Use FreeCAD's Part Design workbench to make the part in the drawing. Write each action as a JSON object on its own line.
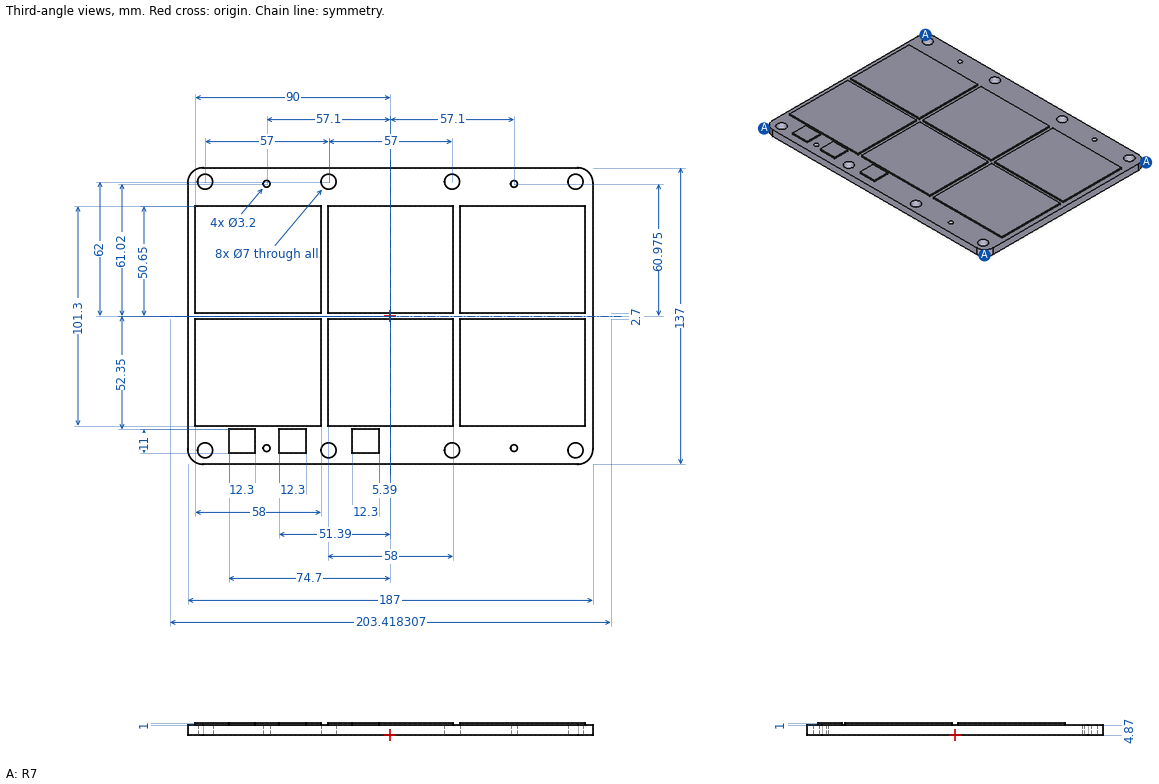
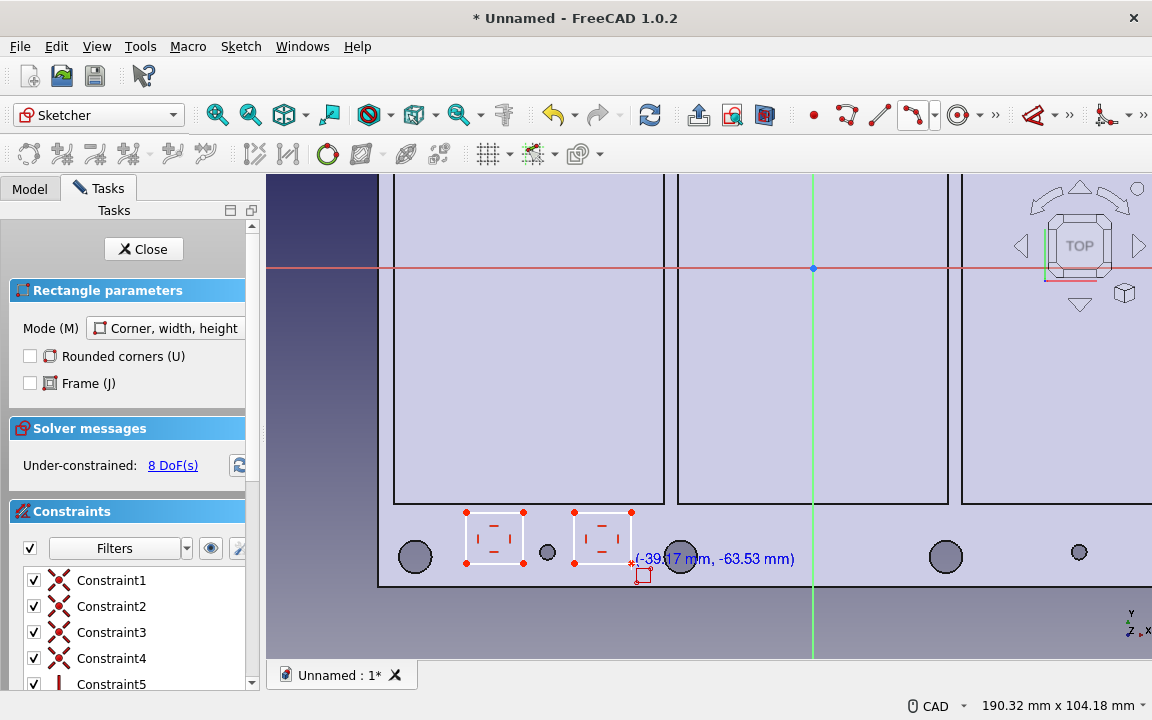
{"action": "left_click", "coordinate": [731, 512]}
{"action": "left_click", "coordinate": [788, 563]}
{"action": "key", "text": "Escape"}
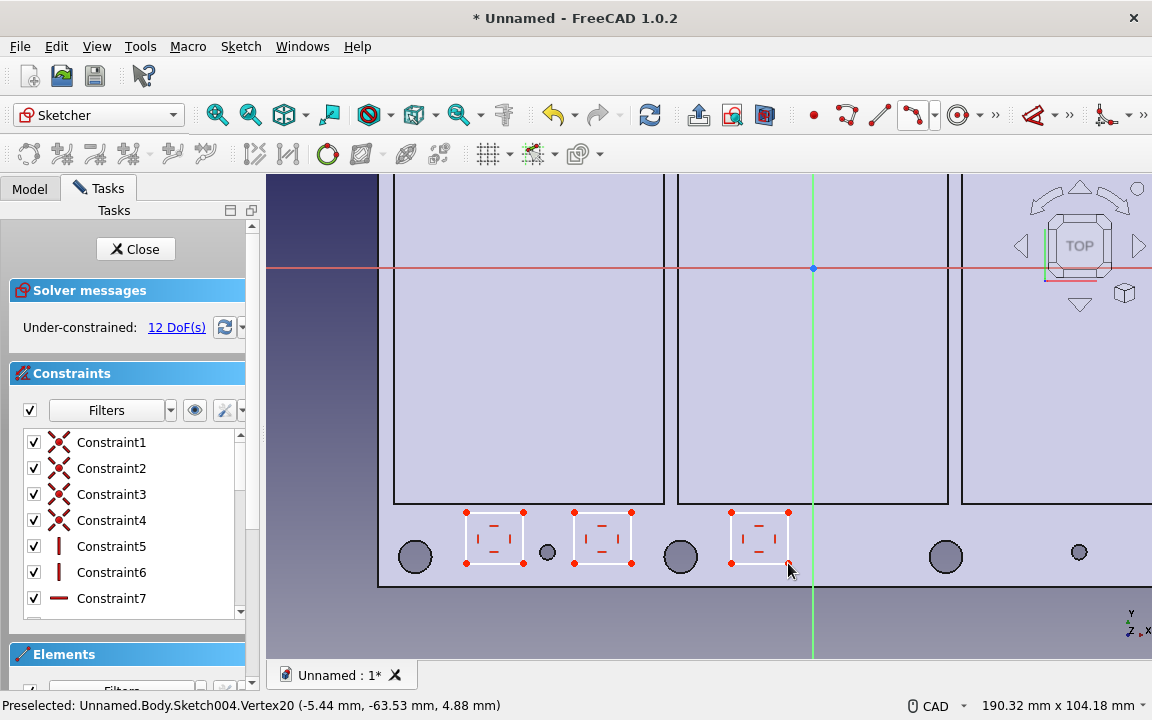
{"action": "key", "text": "d"}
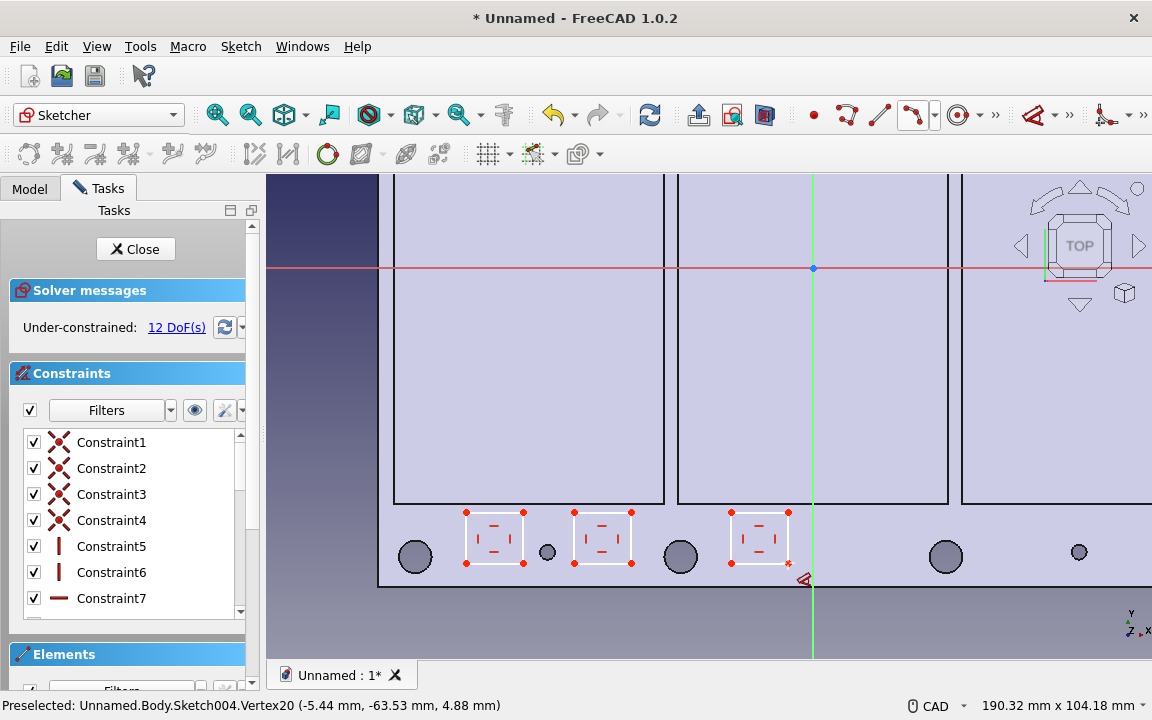
{"action": "left_click", "coordinate": [466, 528]}
{"action": "left_click", "coordinate": [432, 539]}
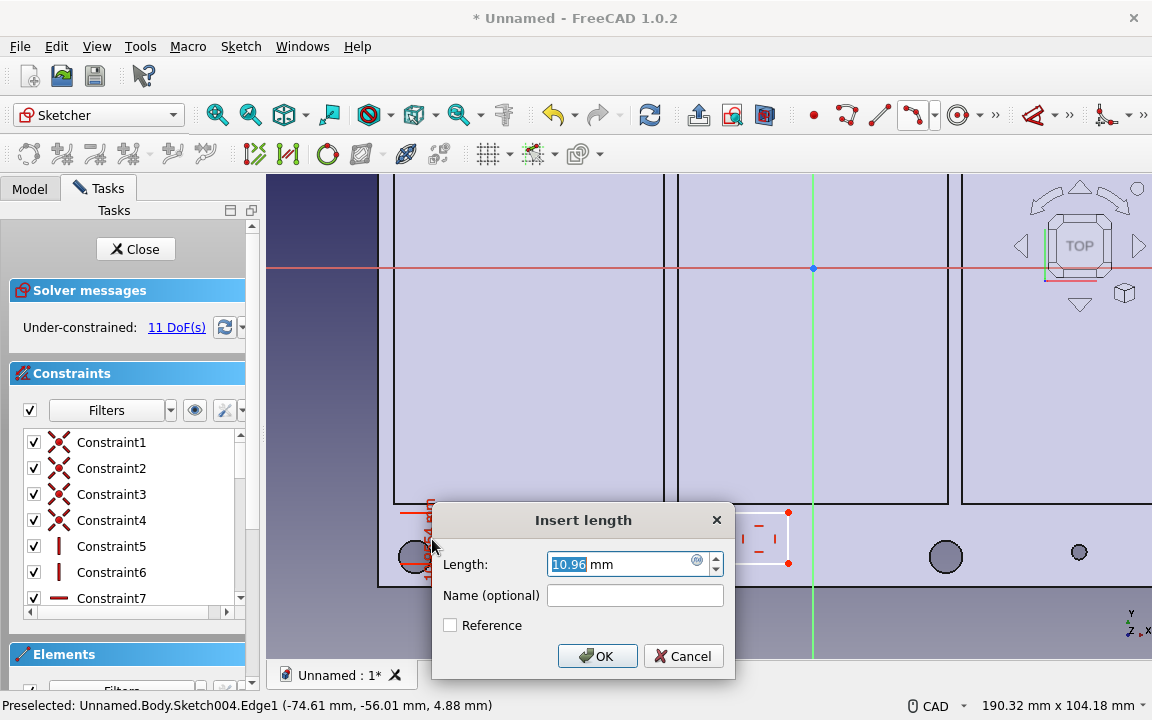
{"action": "type", "text": "11"}
{"action": "key", "text": "Return"}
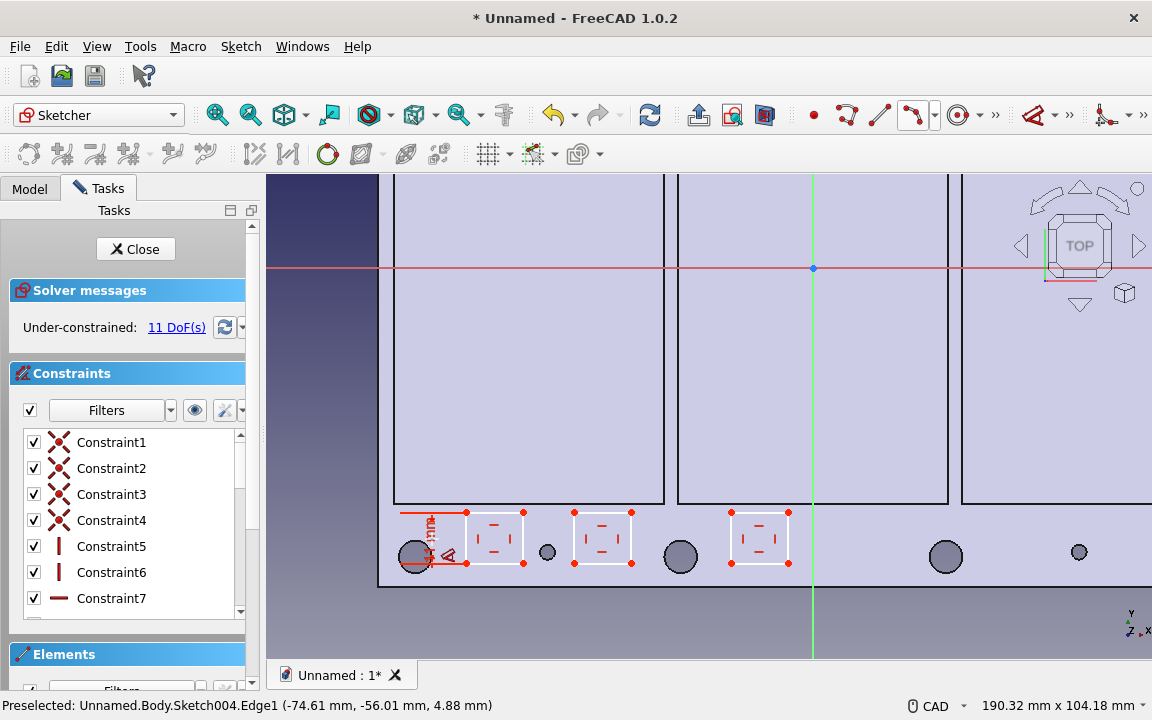
{"action": "left_click", "coordinate": [574, 528]}
{"action": "left_click", "coordinate": [540, 539]}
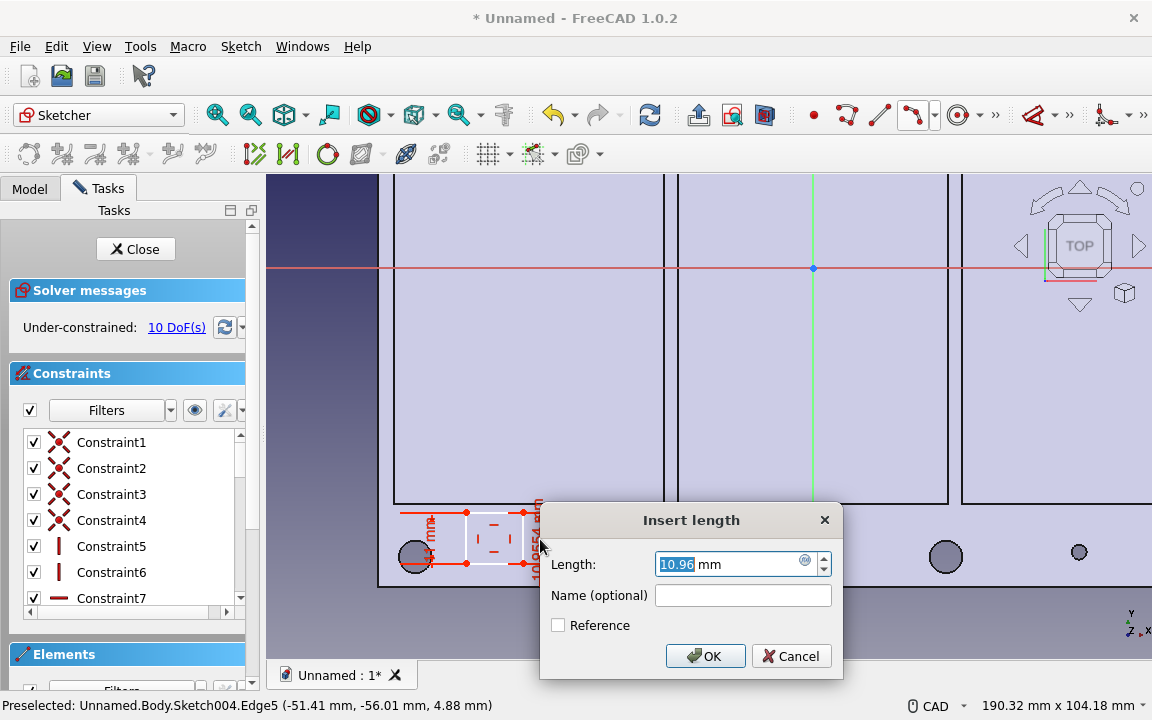
{"action": "type", "text": "11"}
{"action": "key", "text": "Return"}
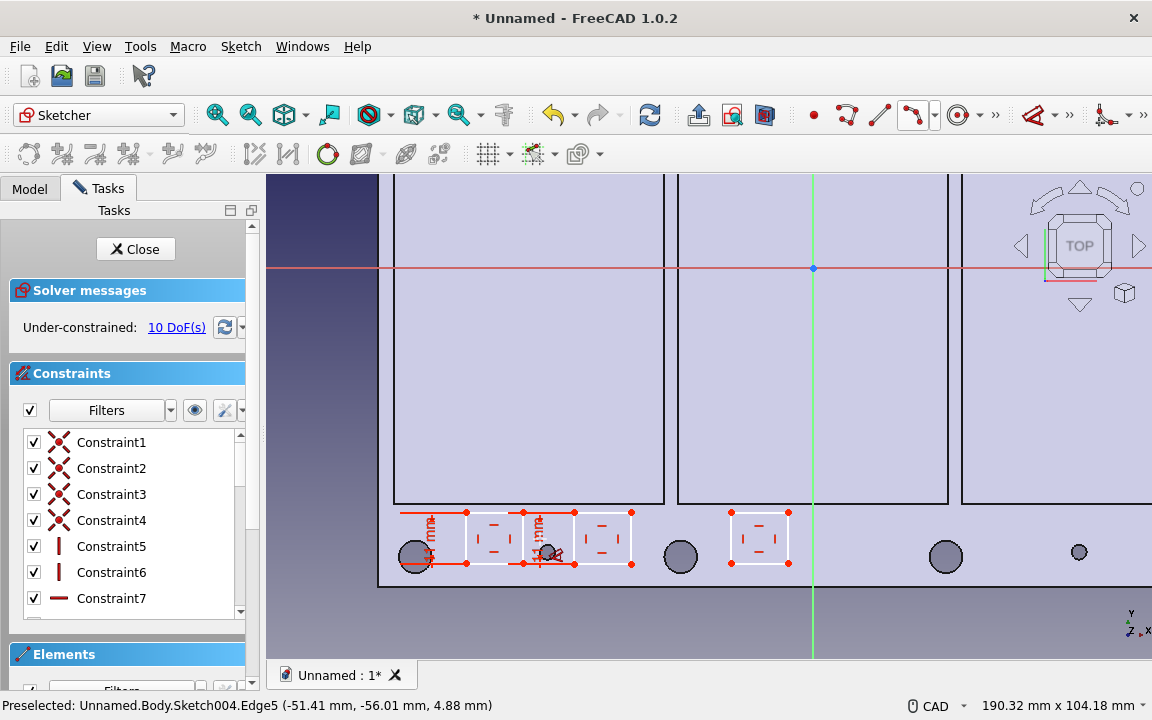
{"action": "left_click", "coordinate": [731, 528]}
{"action": "left_click", "coordinate": [765, 539]}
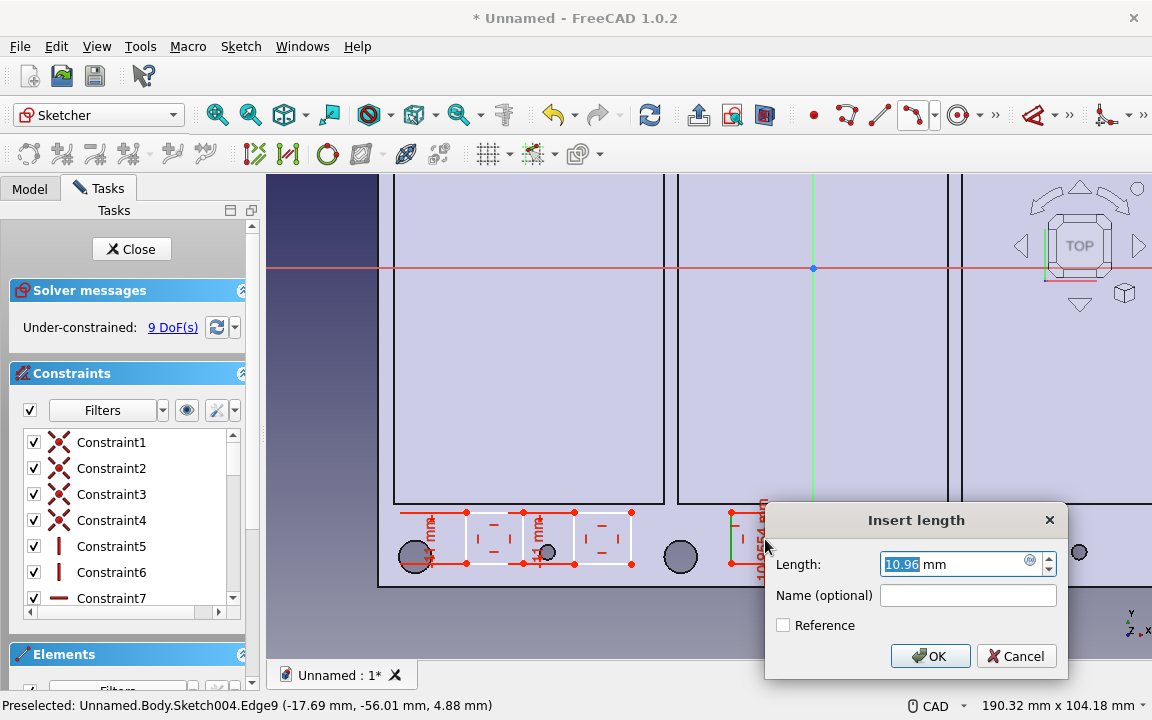
{"action": "type", "text": "11"}
{"action": "key", "text": "Return"}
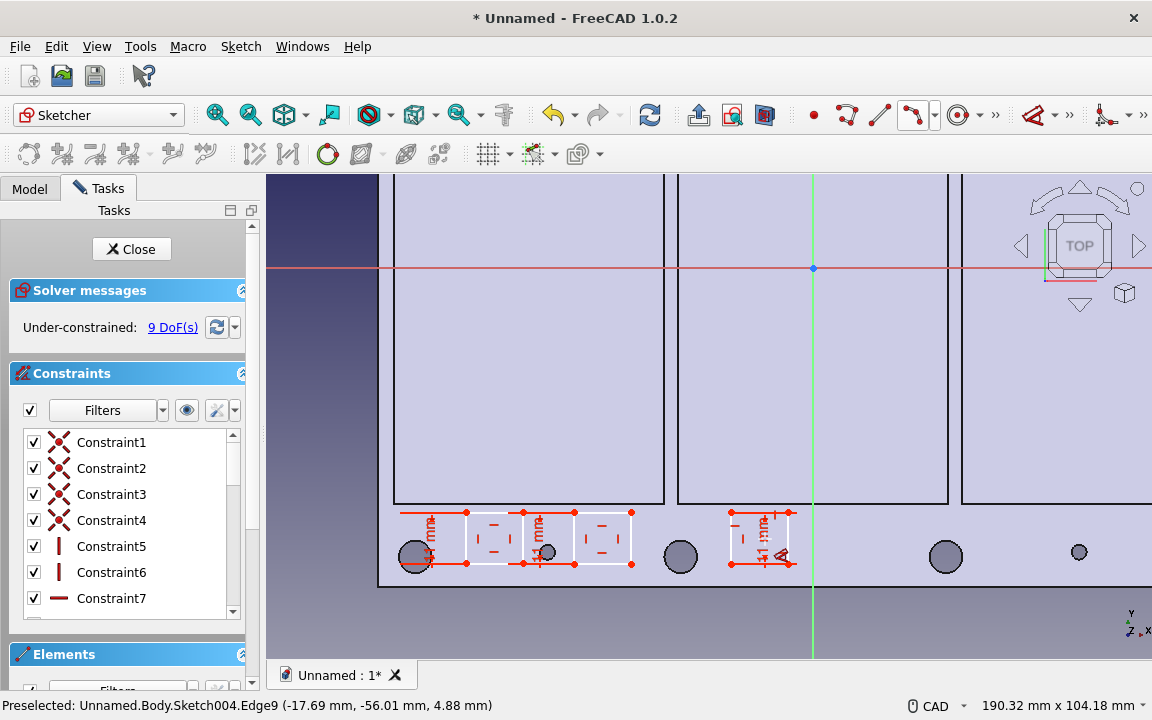
{"action": "left_click", "coordinate": [483, 564]}
{"action": "left_click", "coordinate": [495, 598]}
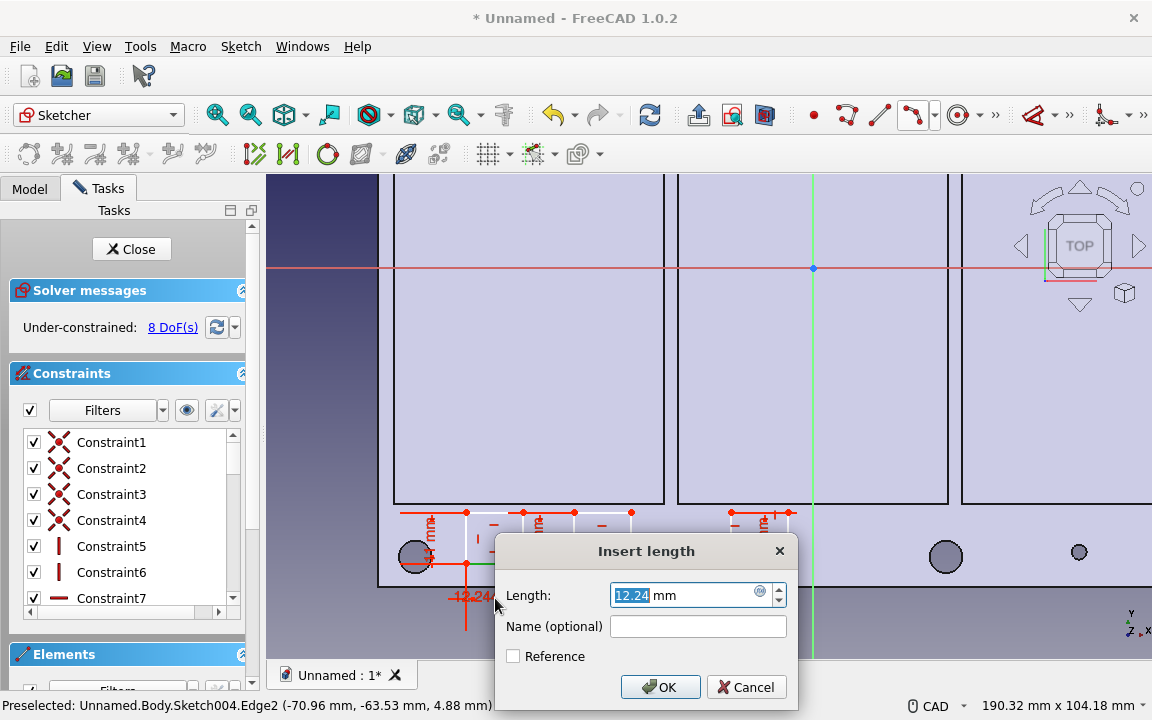
{"action": "type", "text": "12.3"}
{"action": "key", "text": "Return"}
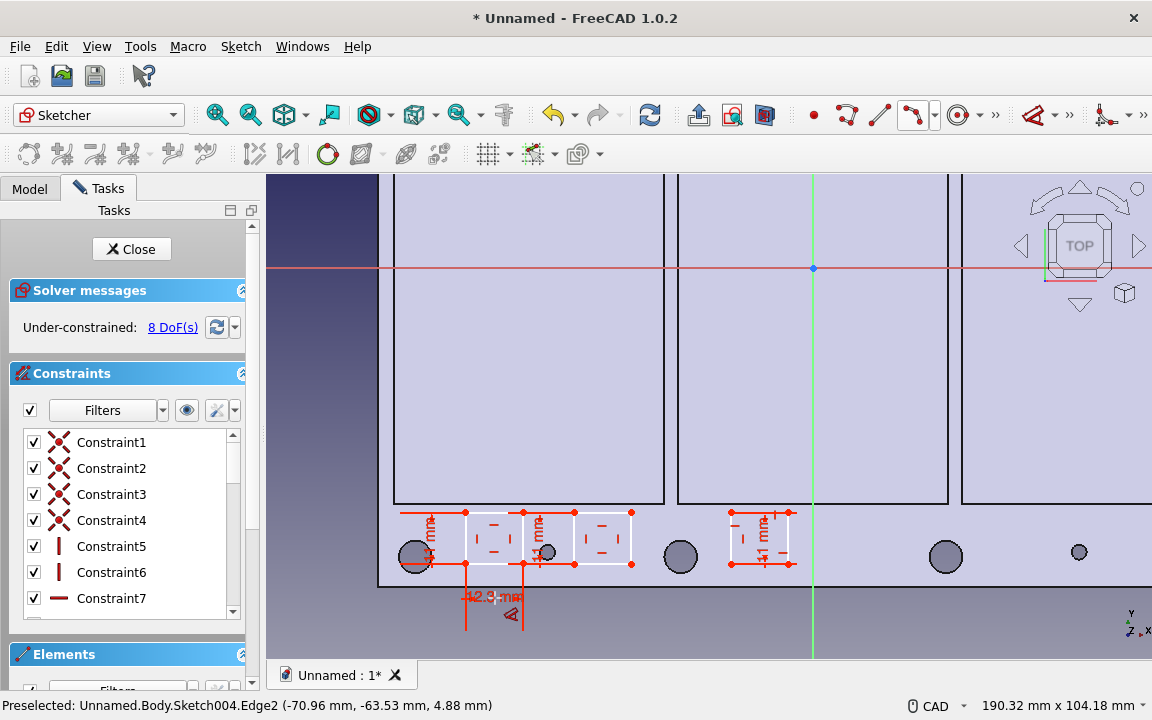
{"action": "left_click", "coordinate": [591, 564]}
{"action": "left_click", "coordinate": [602, 598]}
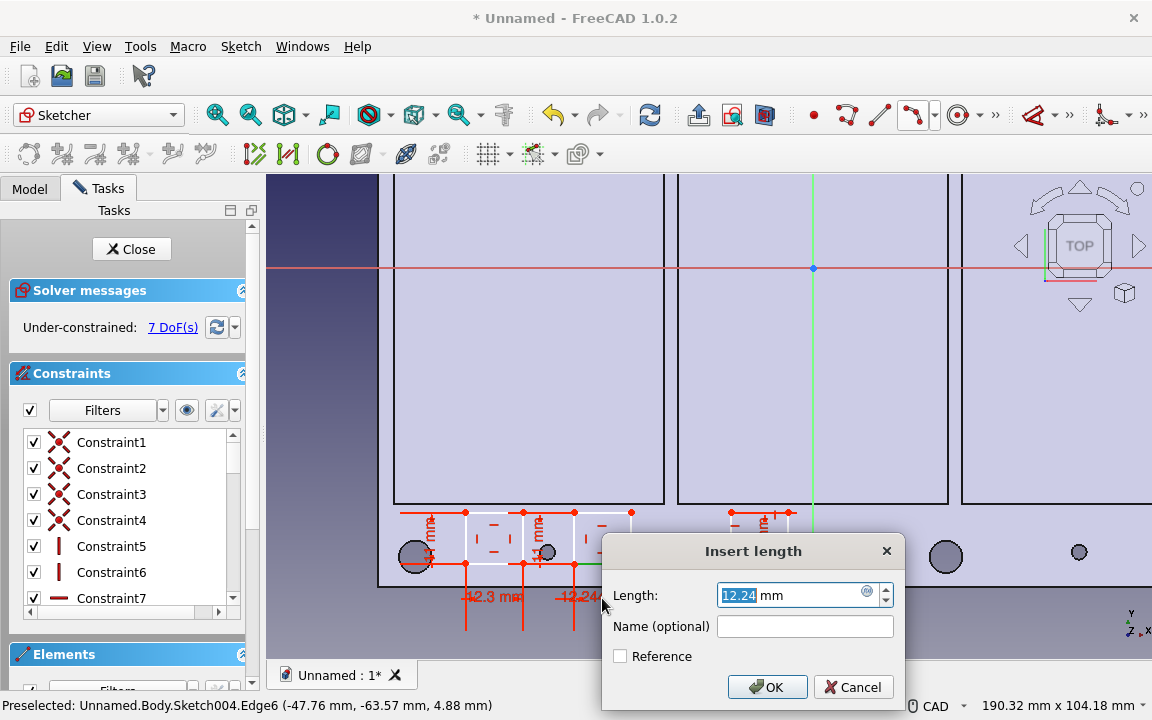
{"action": "type", "text": "12.3"}
{"action": "key", "text": "Return"}